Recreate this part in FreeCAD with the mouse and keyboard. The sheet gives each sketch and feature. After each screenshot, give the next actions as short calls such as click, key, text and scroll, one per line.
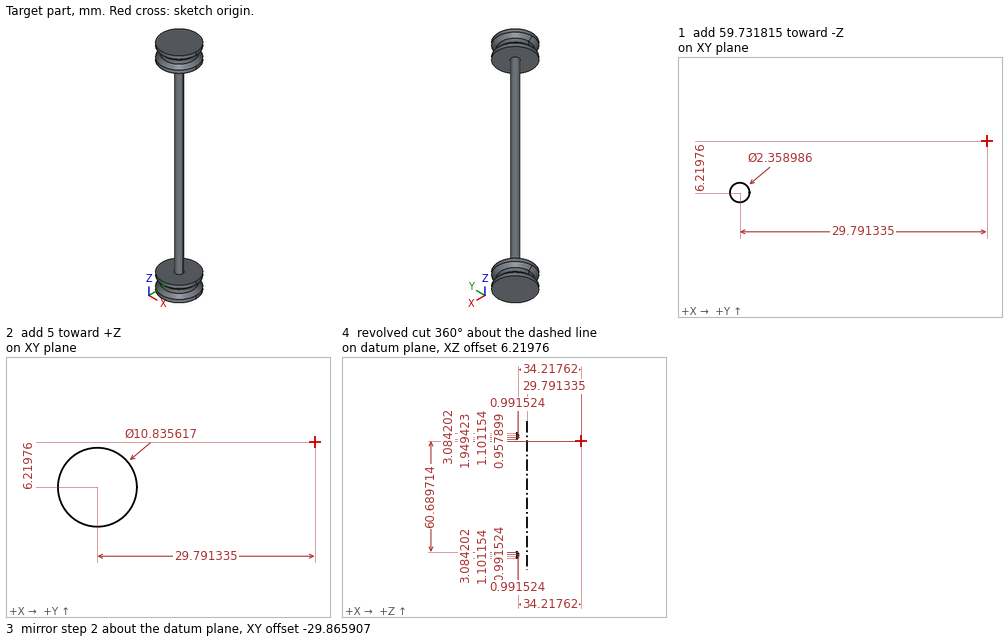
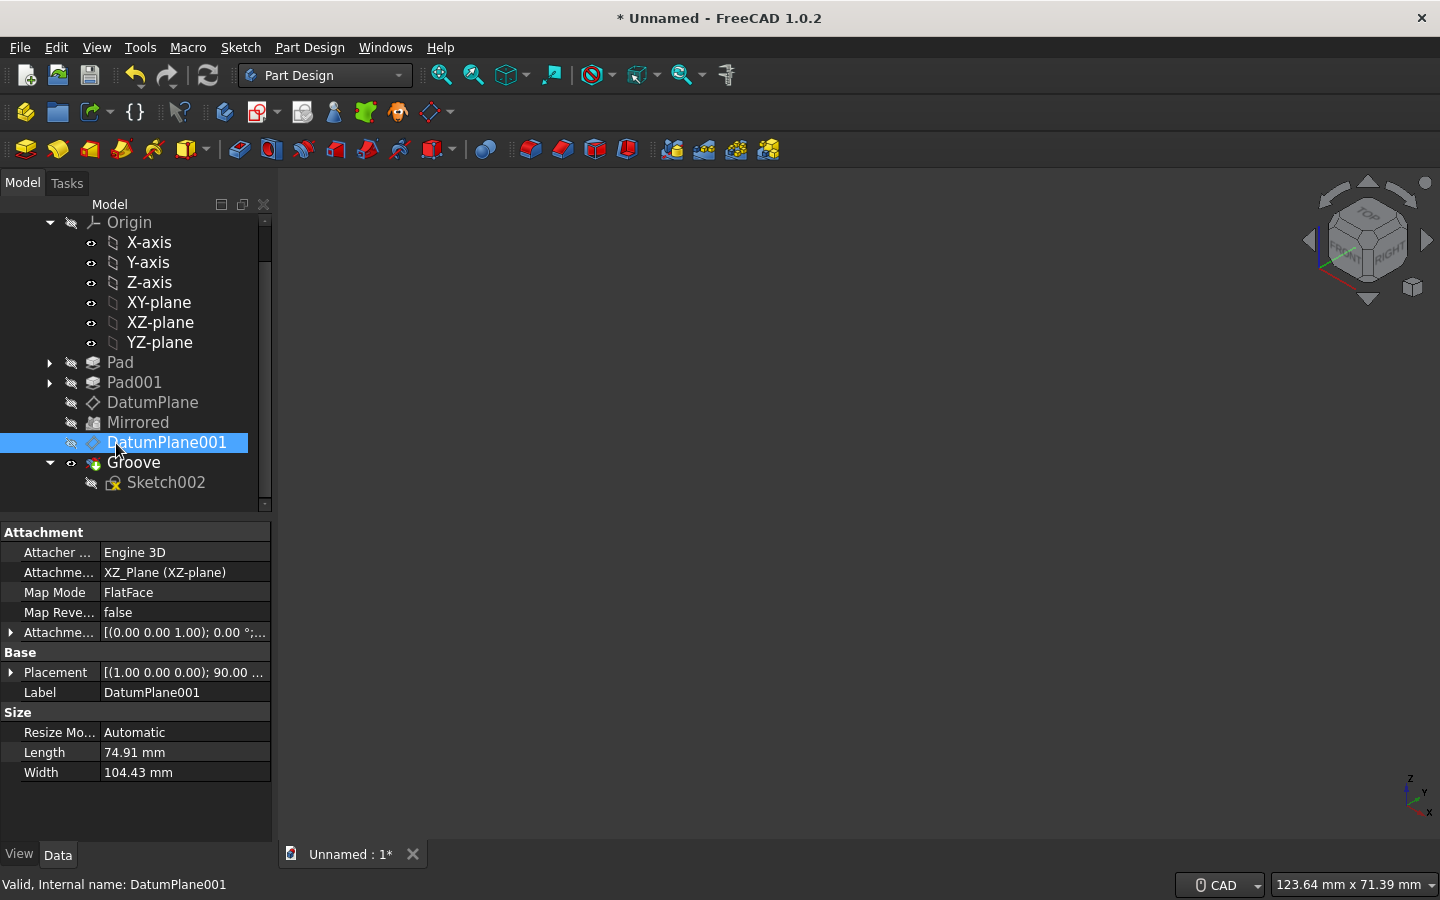
key(v)
key(f)